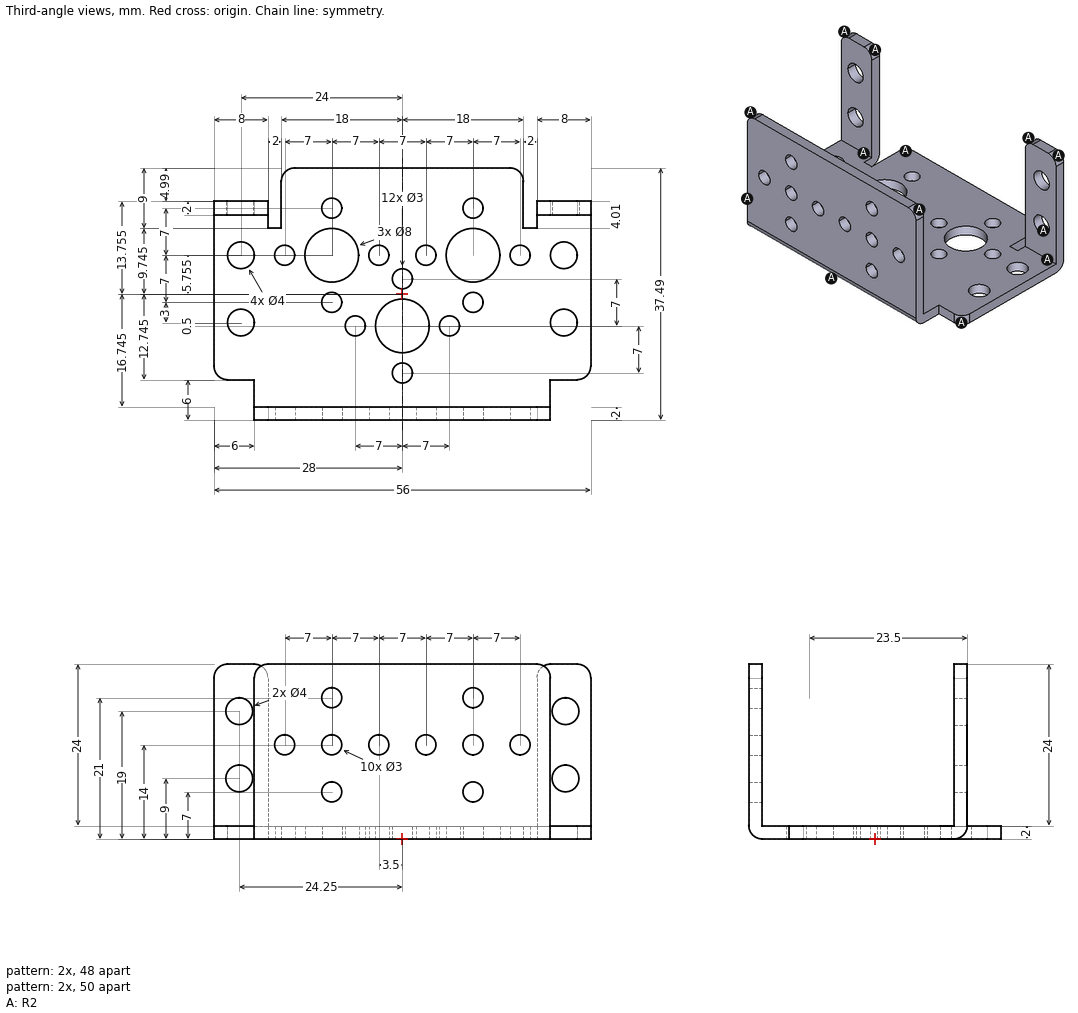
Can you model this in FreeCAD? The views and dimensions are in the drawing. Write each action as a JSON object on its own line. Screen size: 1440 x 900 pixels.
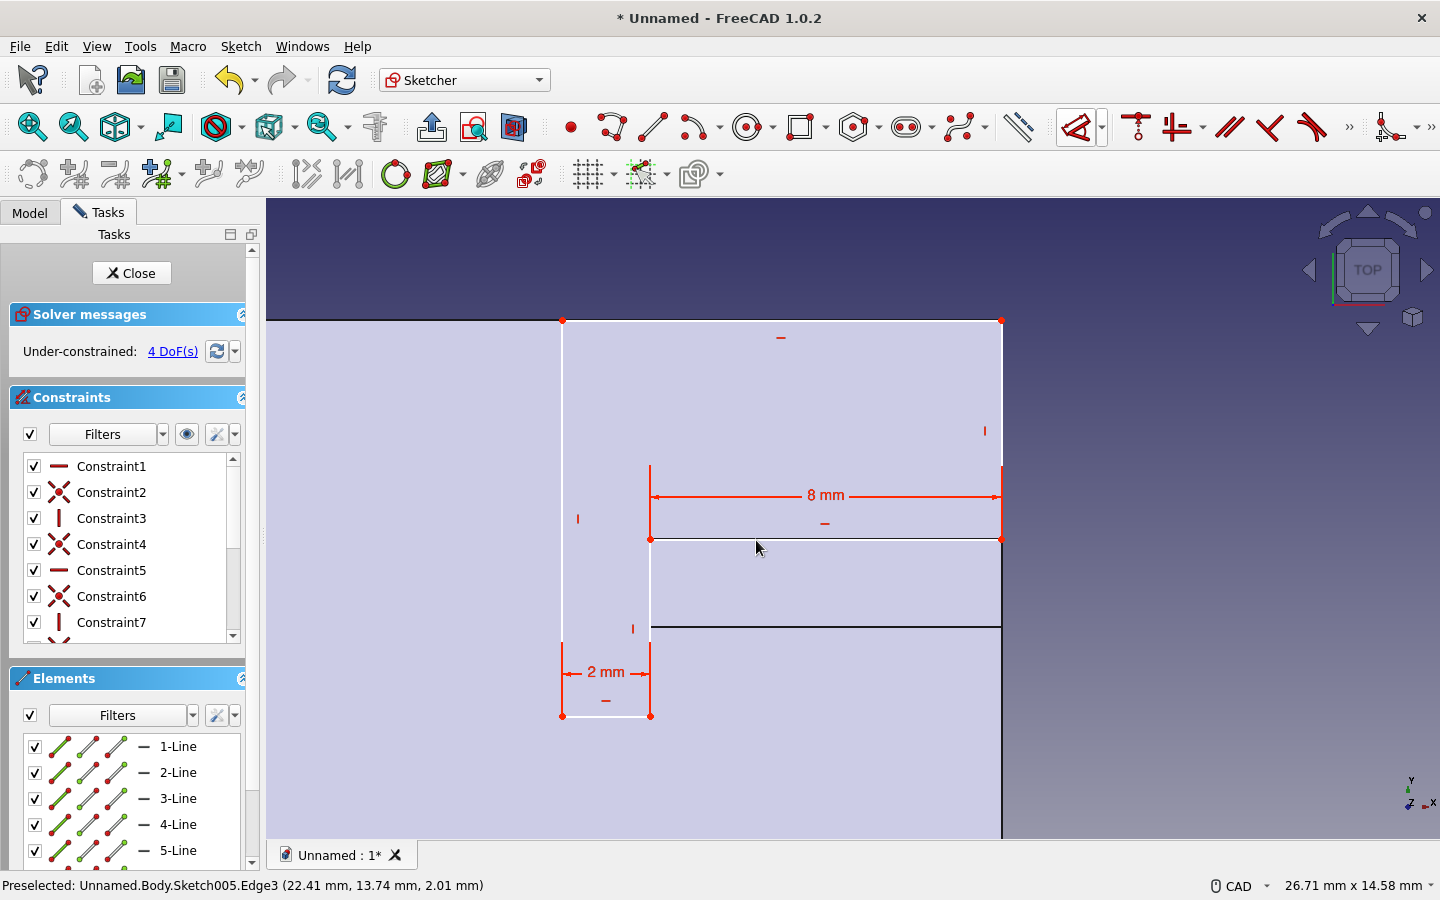
{"action": "left_click", "coordinate": [562, 440]}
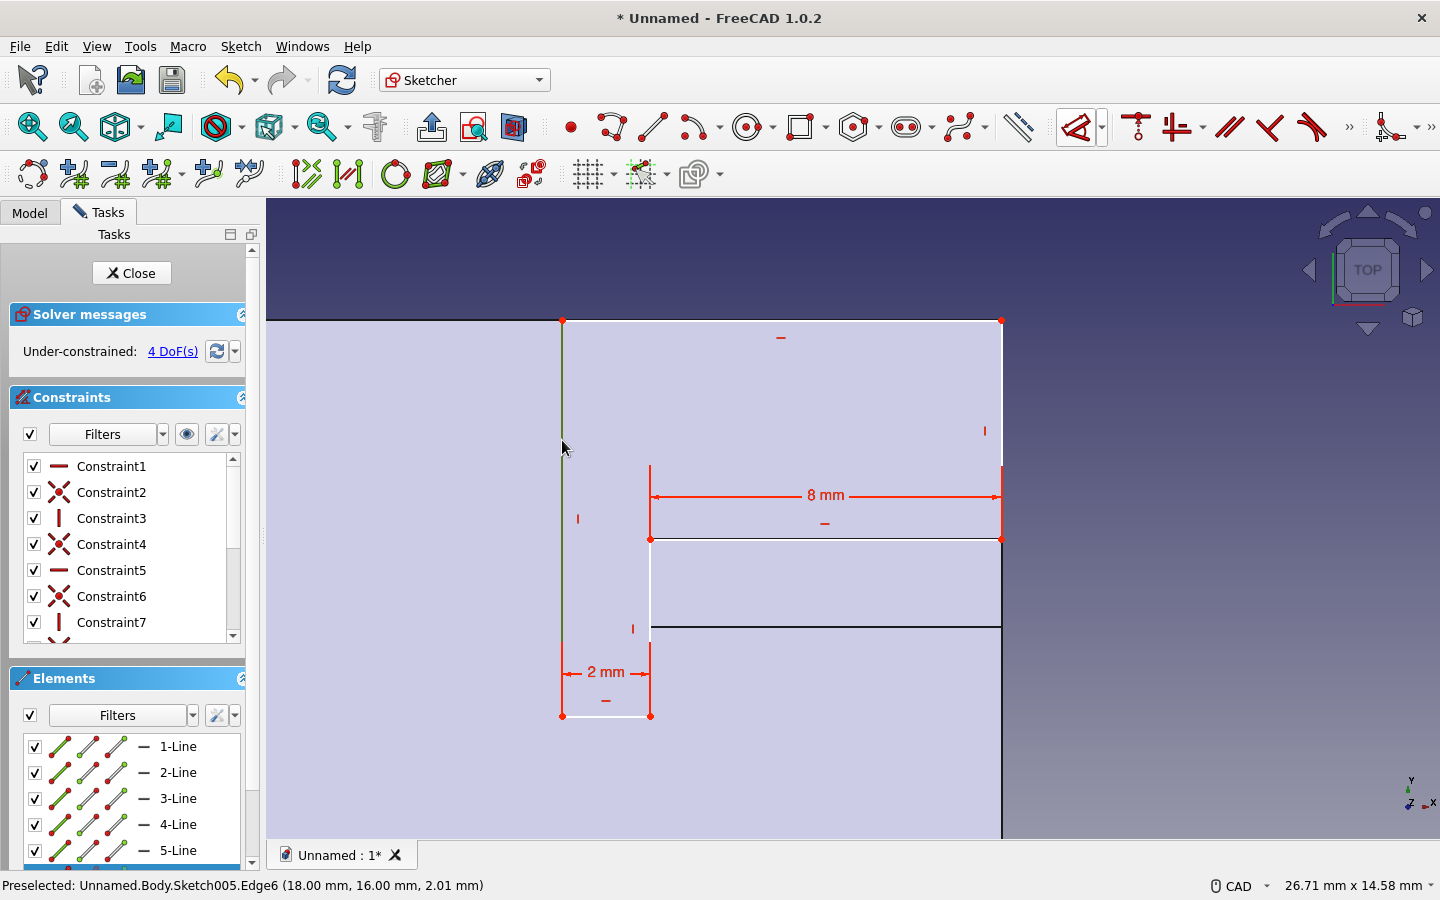
{"action": "key", "text": "i"}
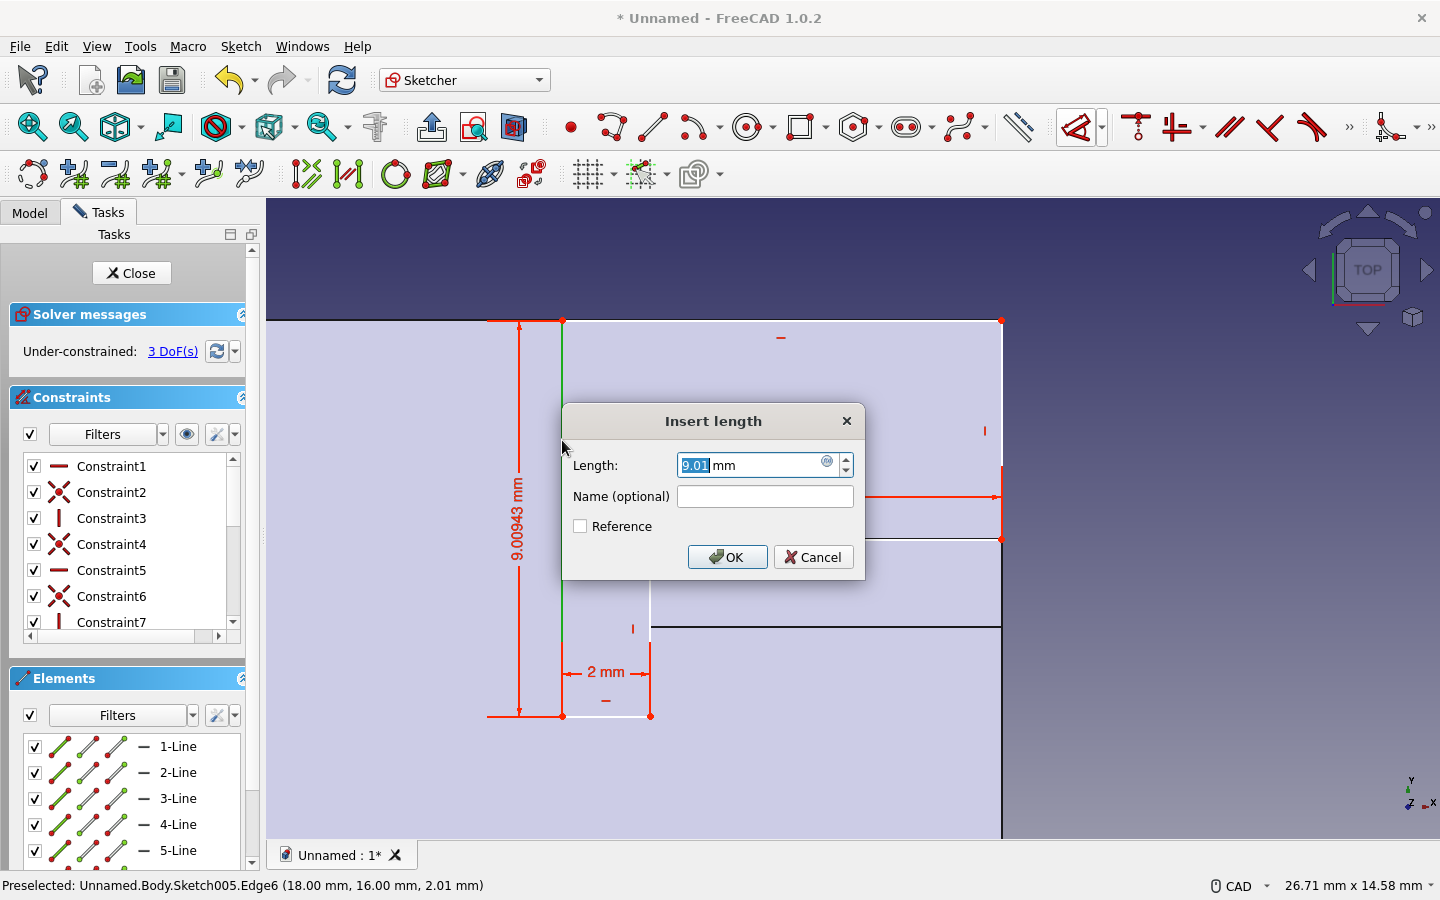
{"action": "type", "text": "9"}
{"action": "key", "text": "Return"}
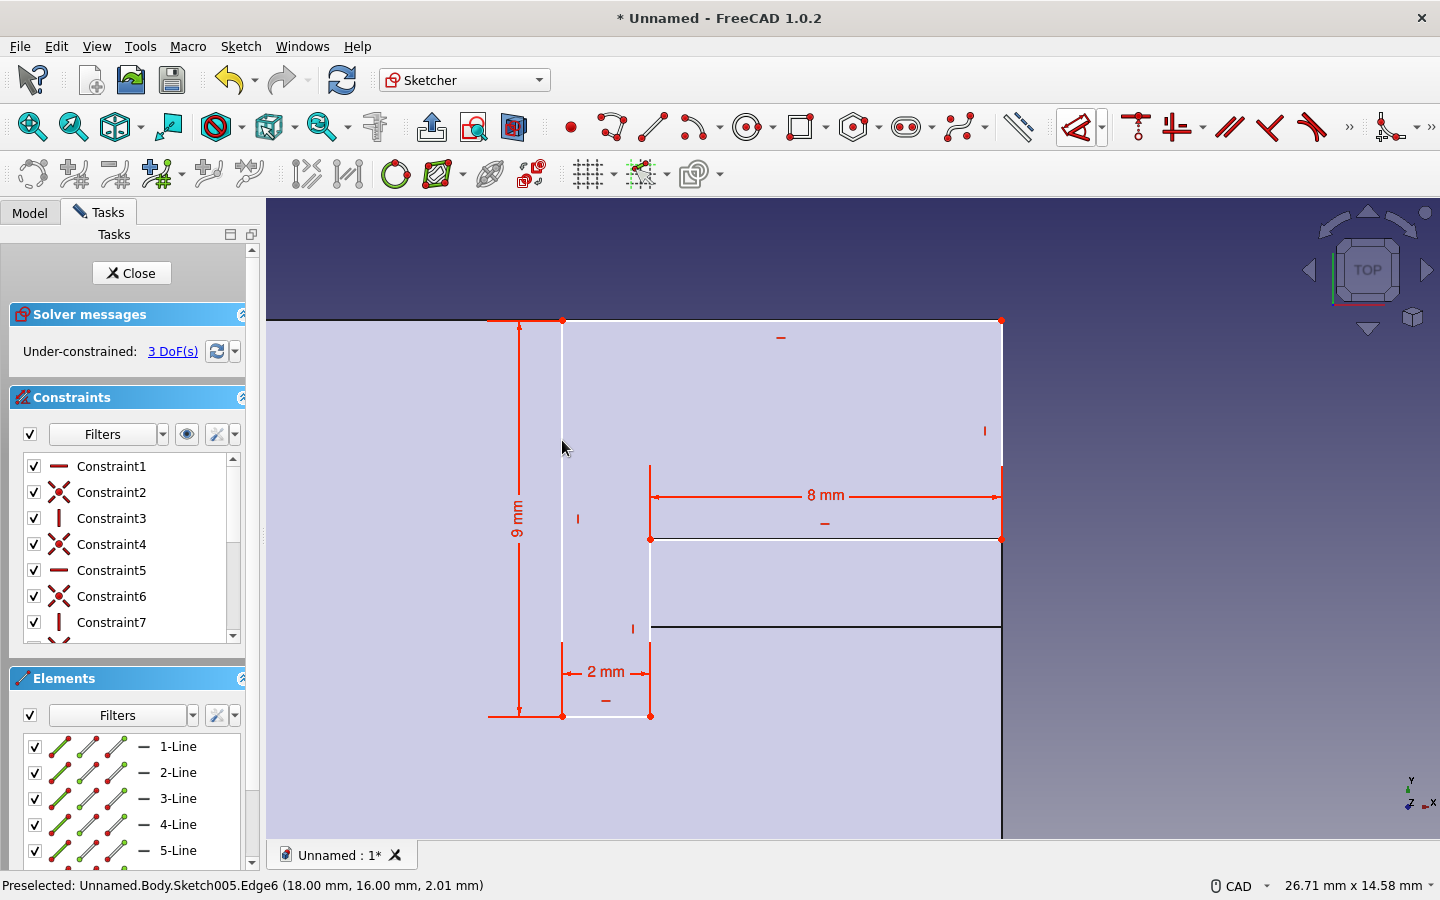
{"action": "left_click", "coordinate": [562, 717]}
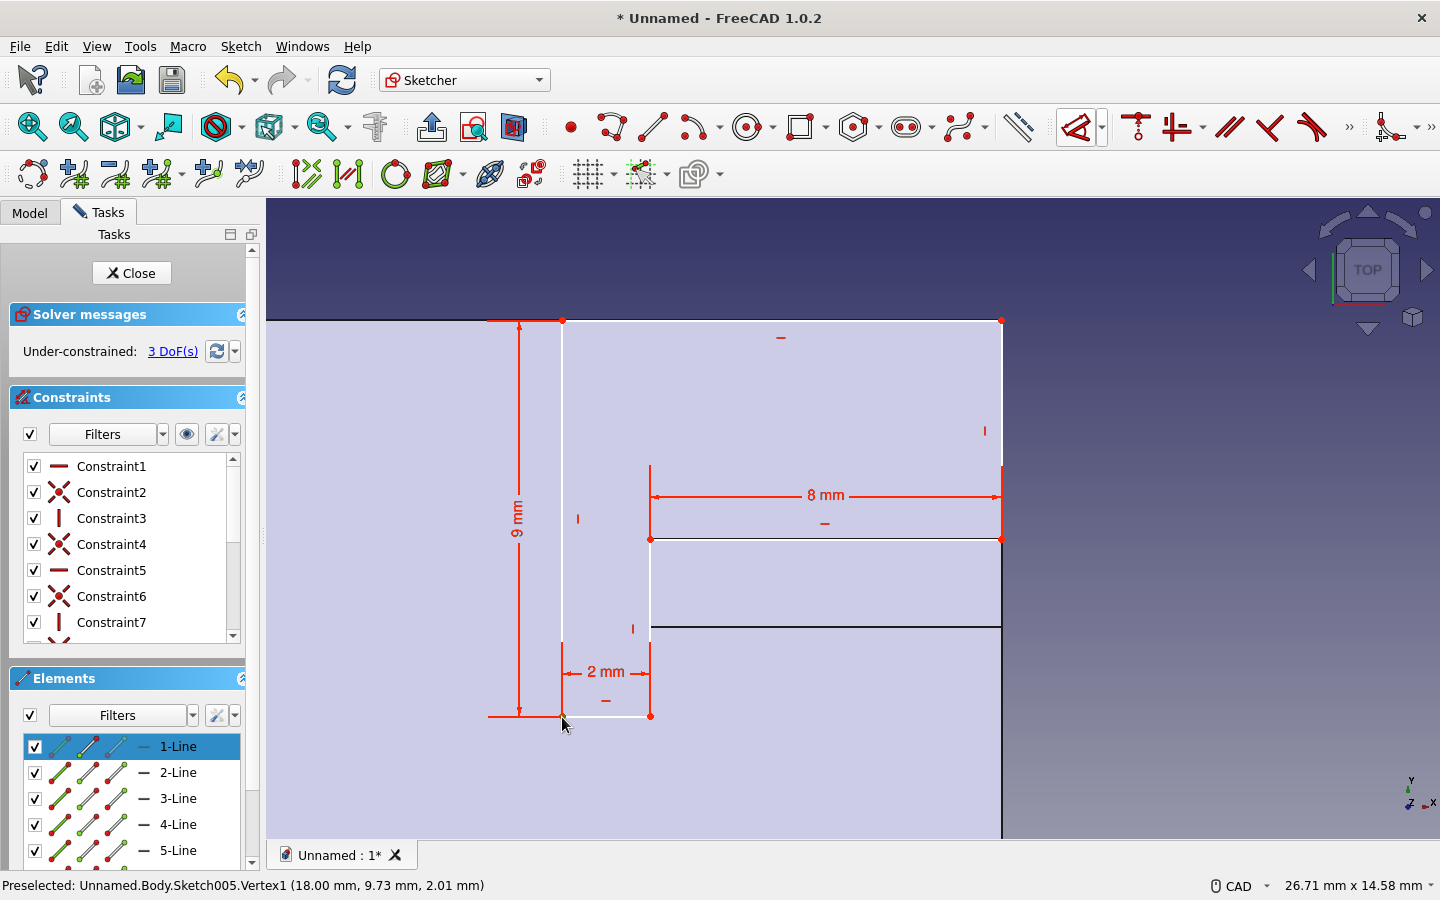
{"action": "key", "text": "l"}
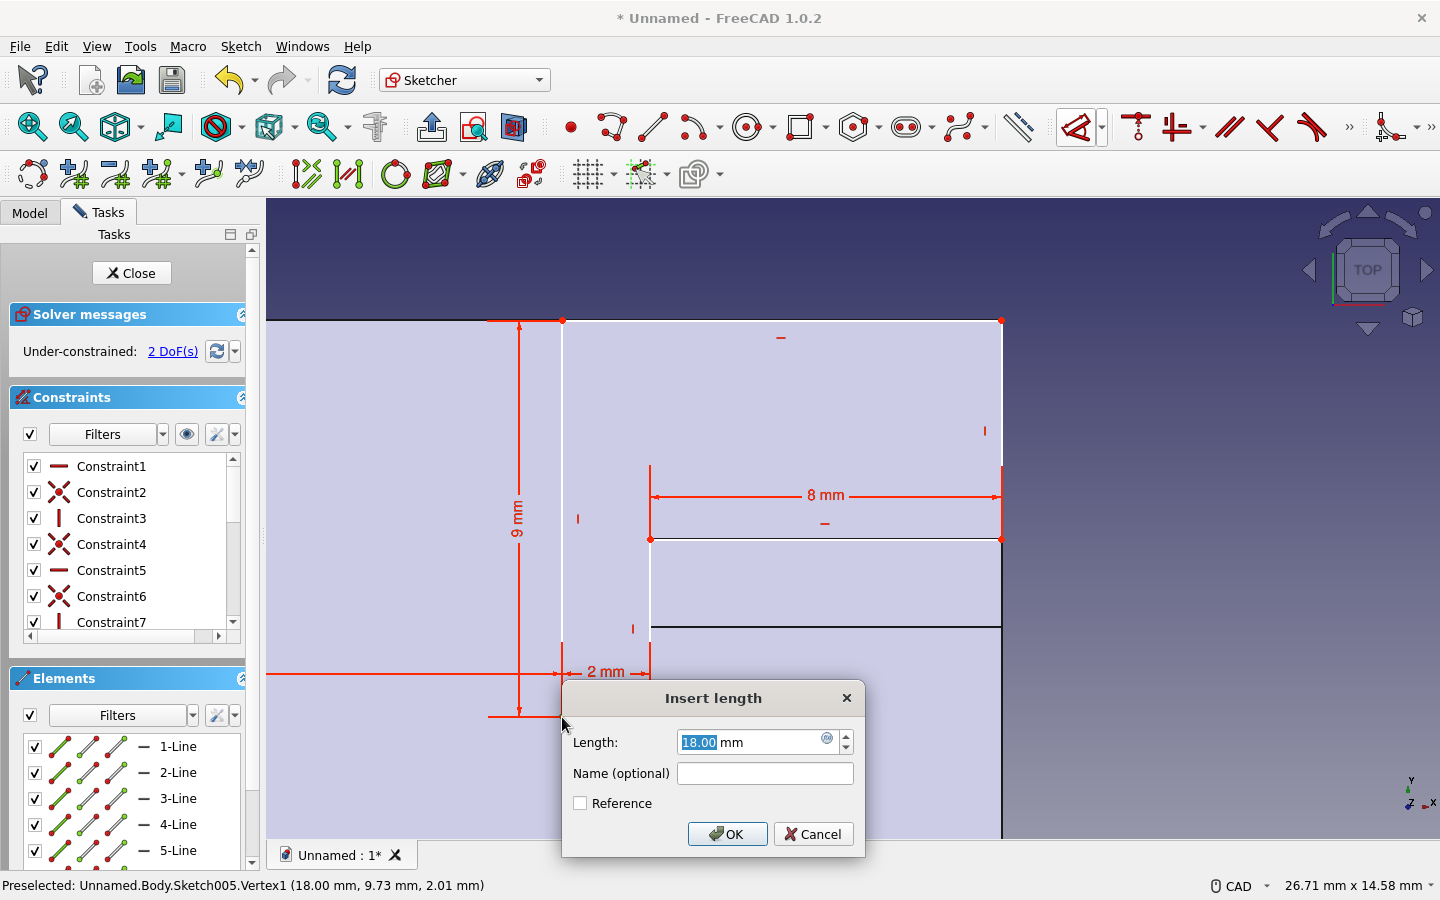
{"action": "type", "text": "18"}
{"action": "key", "text": "Return"}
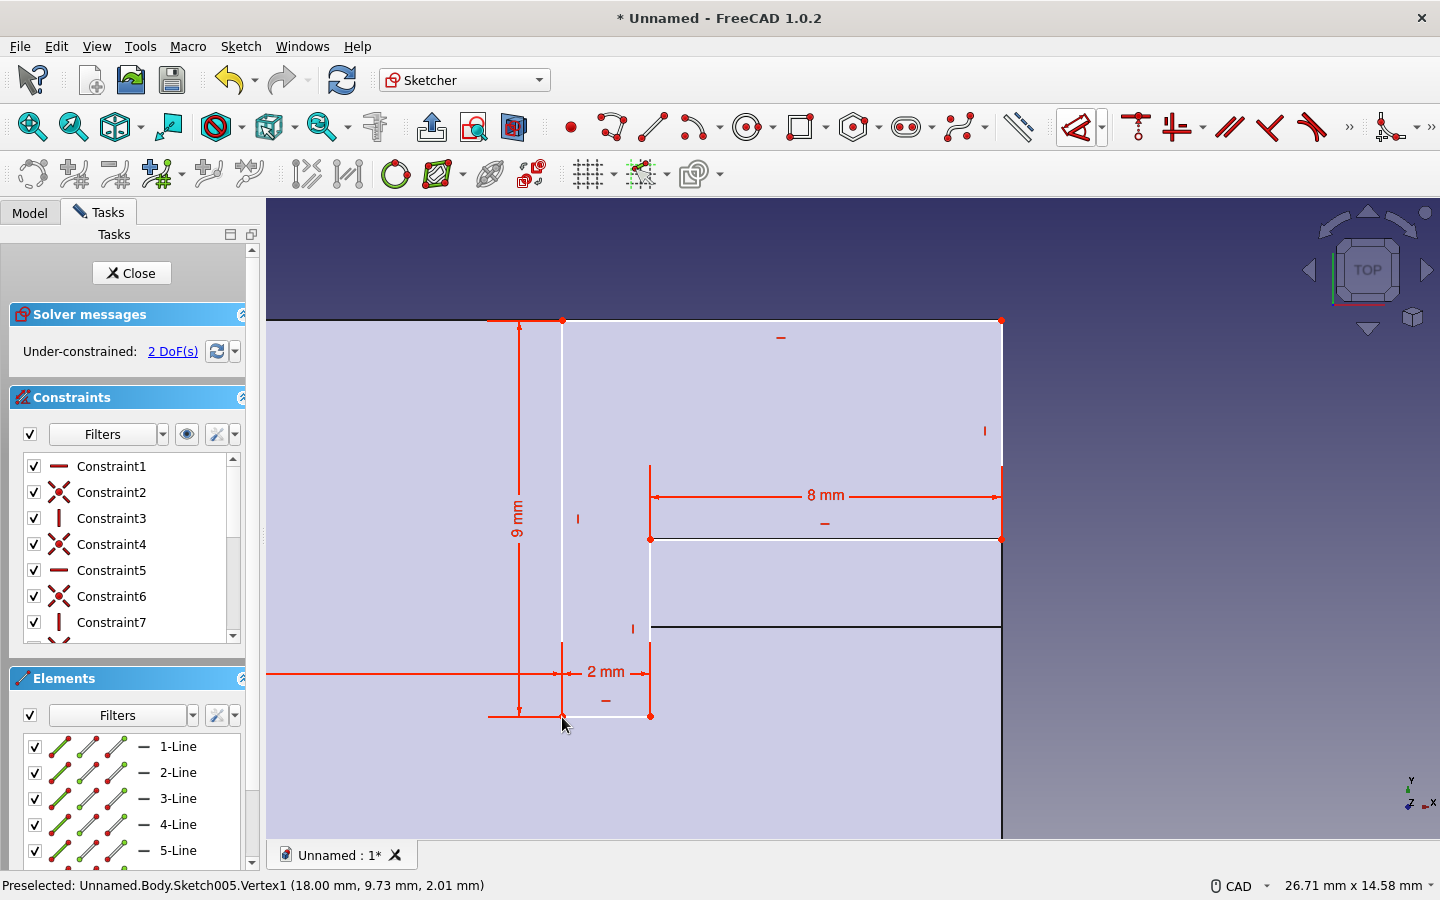
{"action": "left_click", "coordinate": [650, 664]}